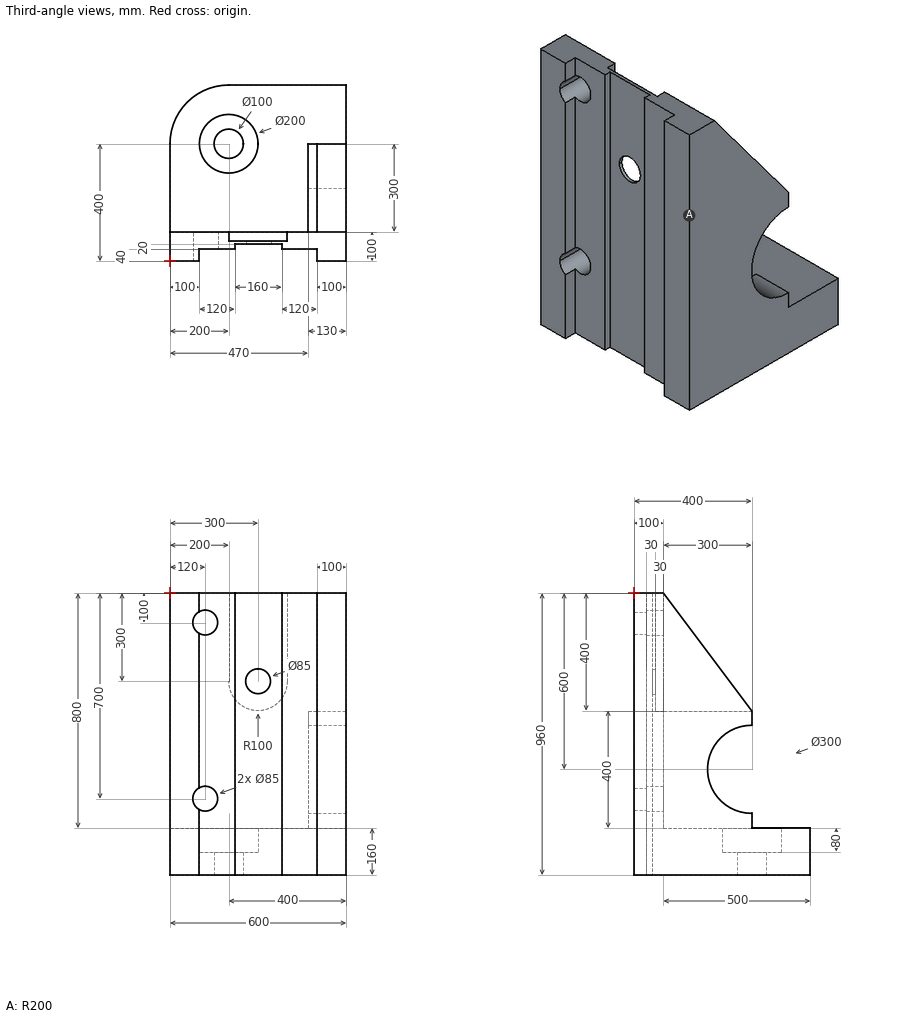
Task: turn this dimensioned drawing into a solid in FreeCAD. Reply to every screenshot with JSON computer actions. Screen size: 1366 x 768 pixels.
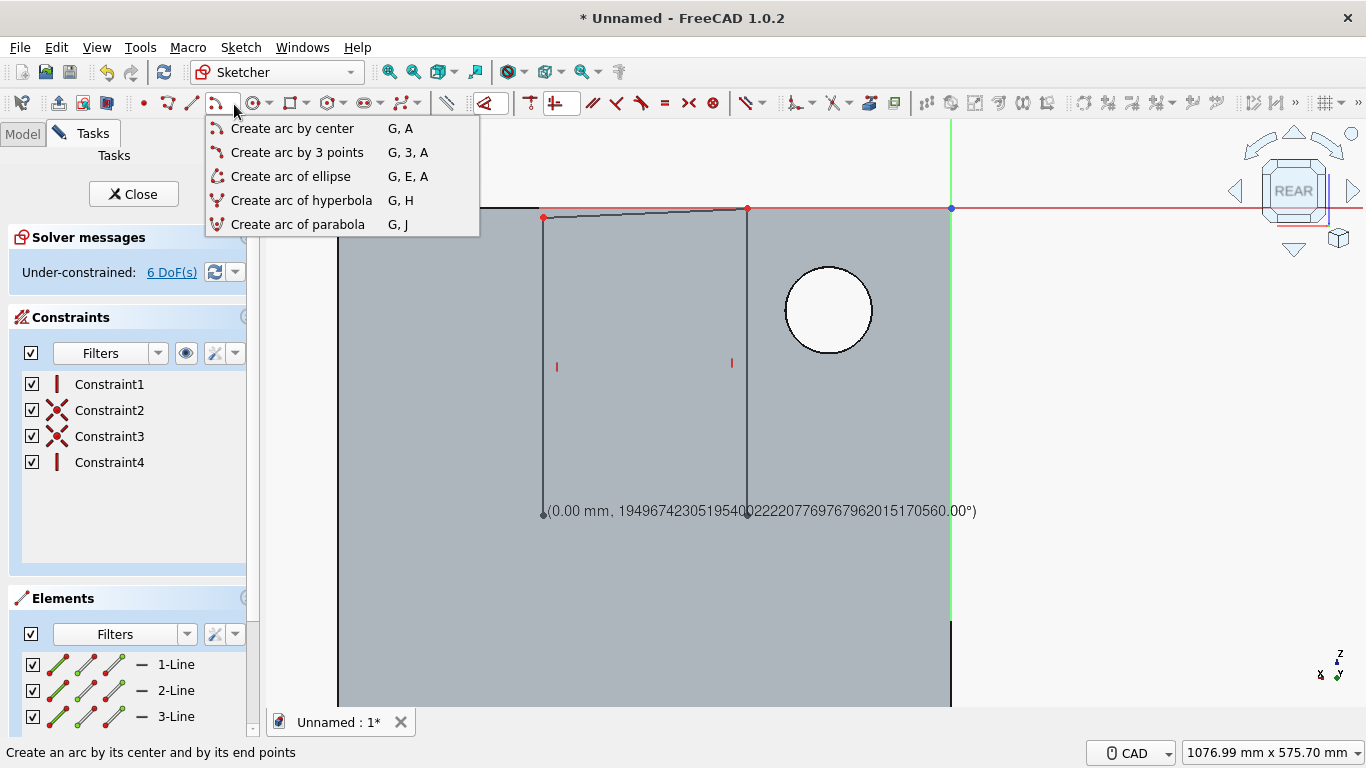
{"action": "left_click", "coordinate": [342, 152]}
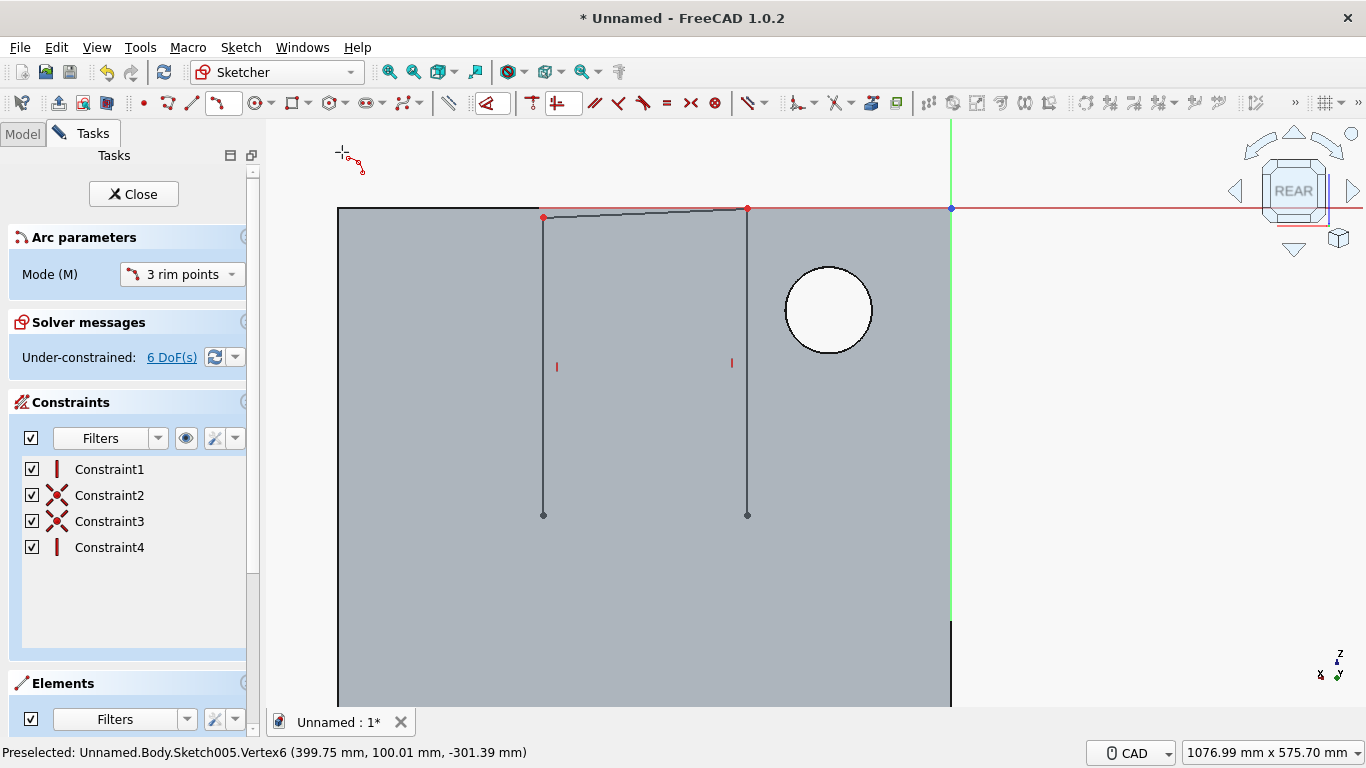
{"action": "left_click", "coordinate": [543, 516]}
{"action": "left_click", "coordinate": [747, 516]}
{"action": "left_click", "coordinate": [645, 617]}
{"action": "key", "text": "Escape"}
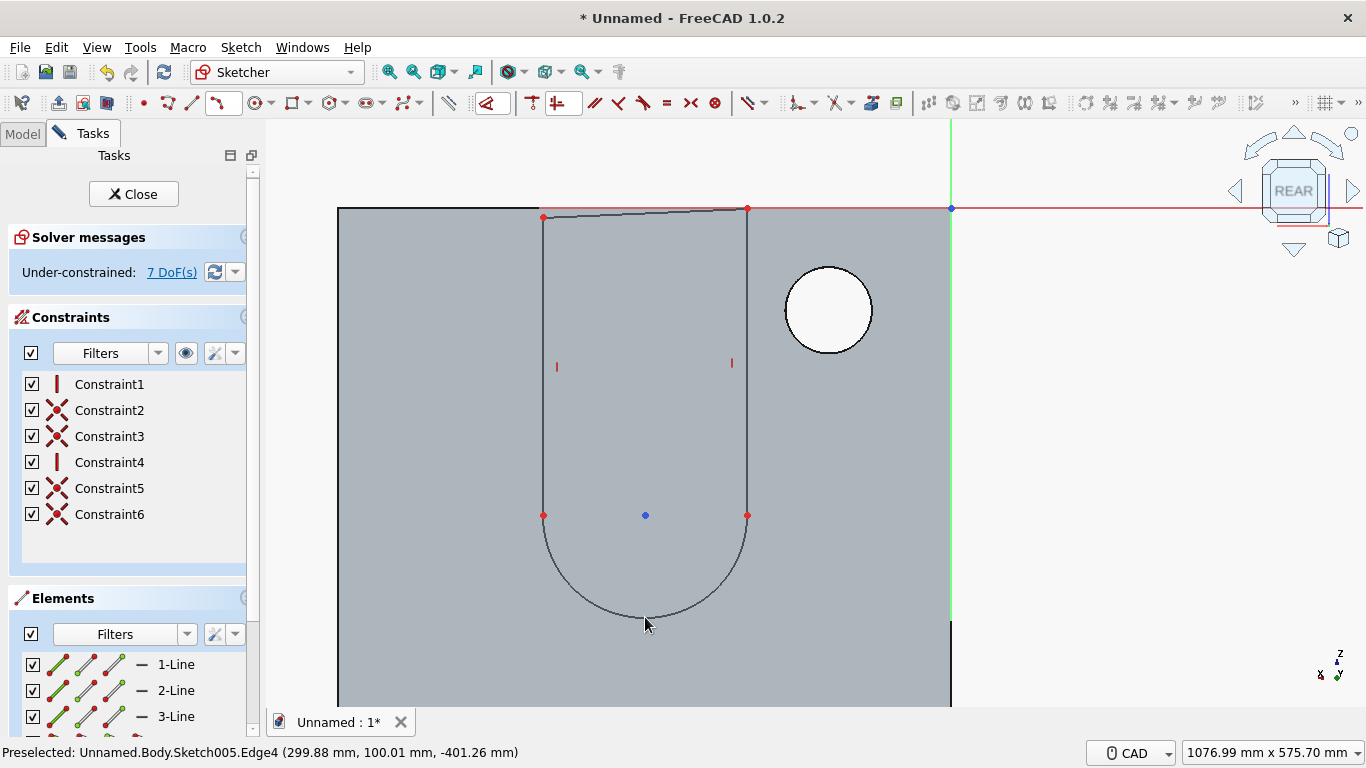
{"action": "left_click", "coordinate": [686, 212]}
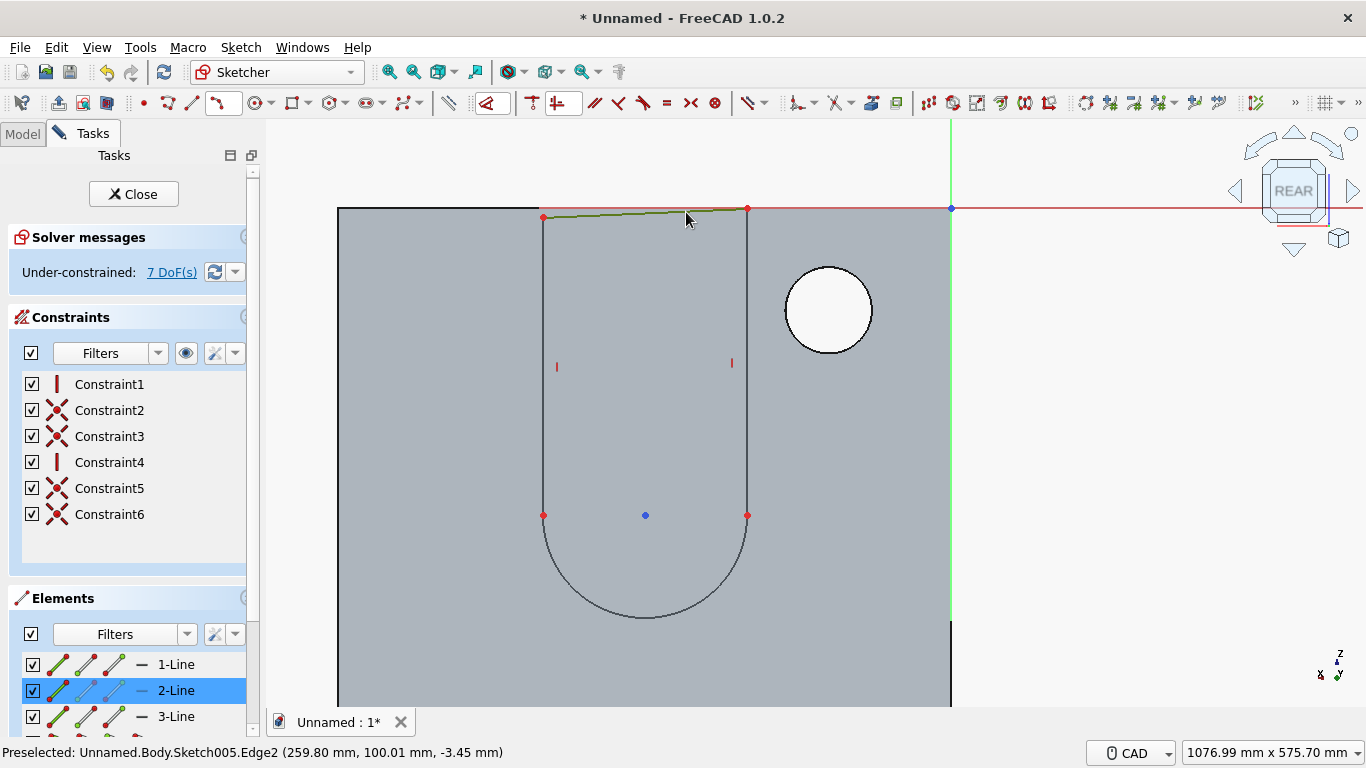
{"action": "key", "text": "h"}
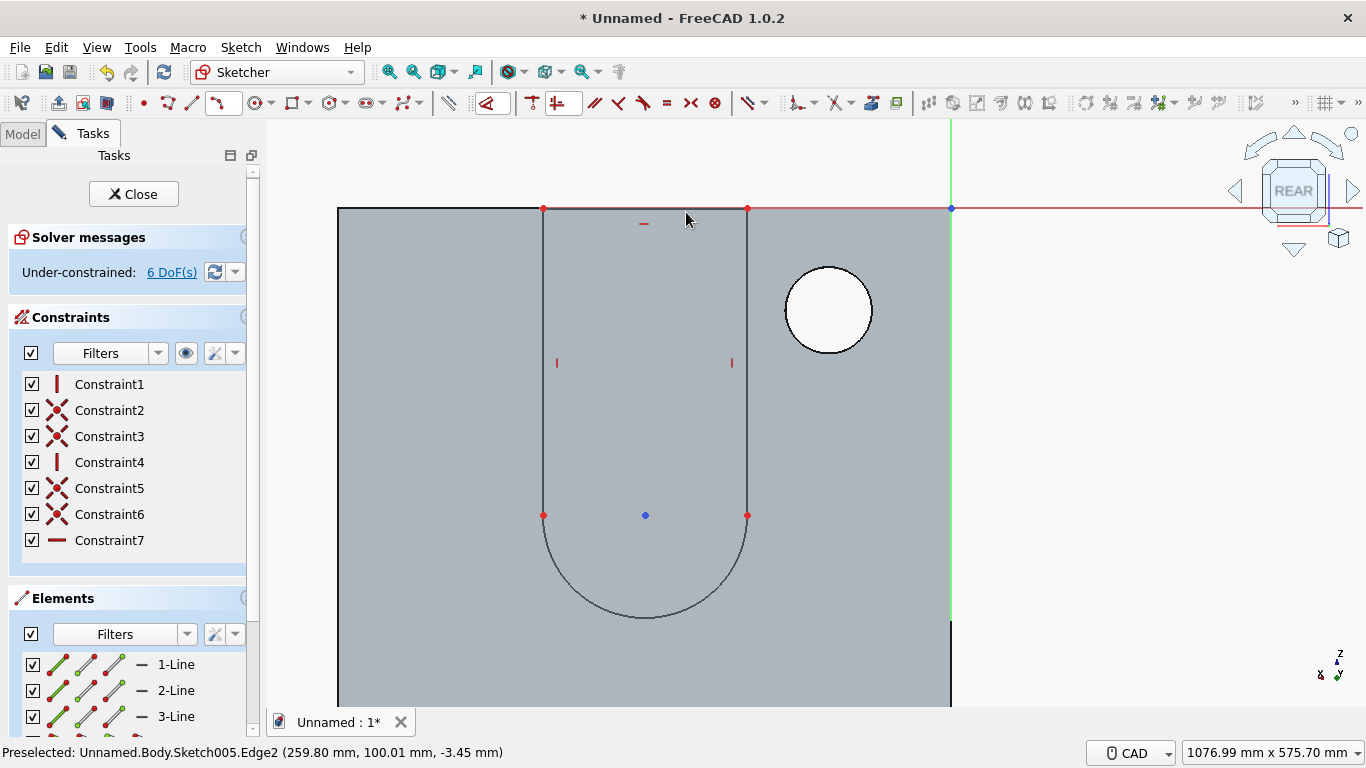
{"action": "left_click", "coordinate": [585, 599]}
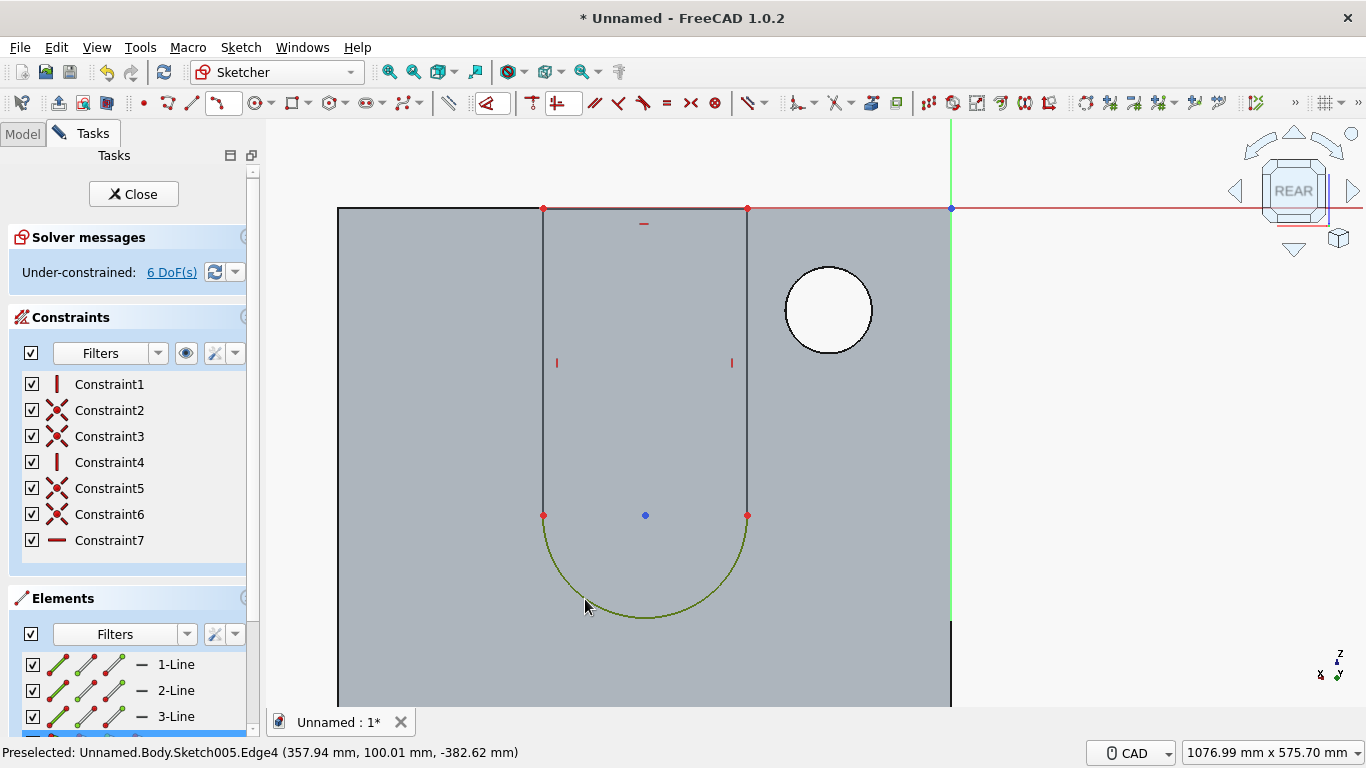
{"action": "left_click", "coordinate": [504, 104]}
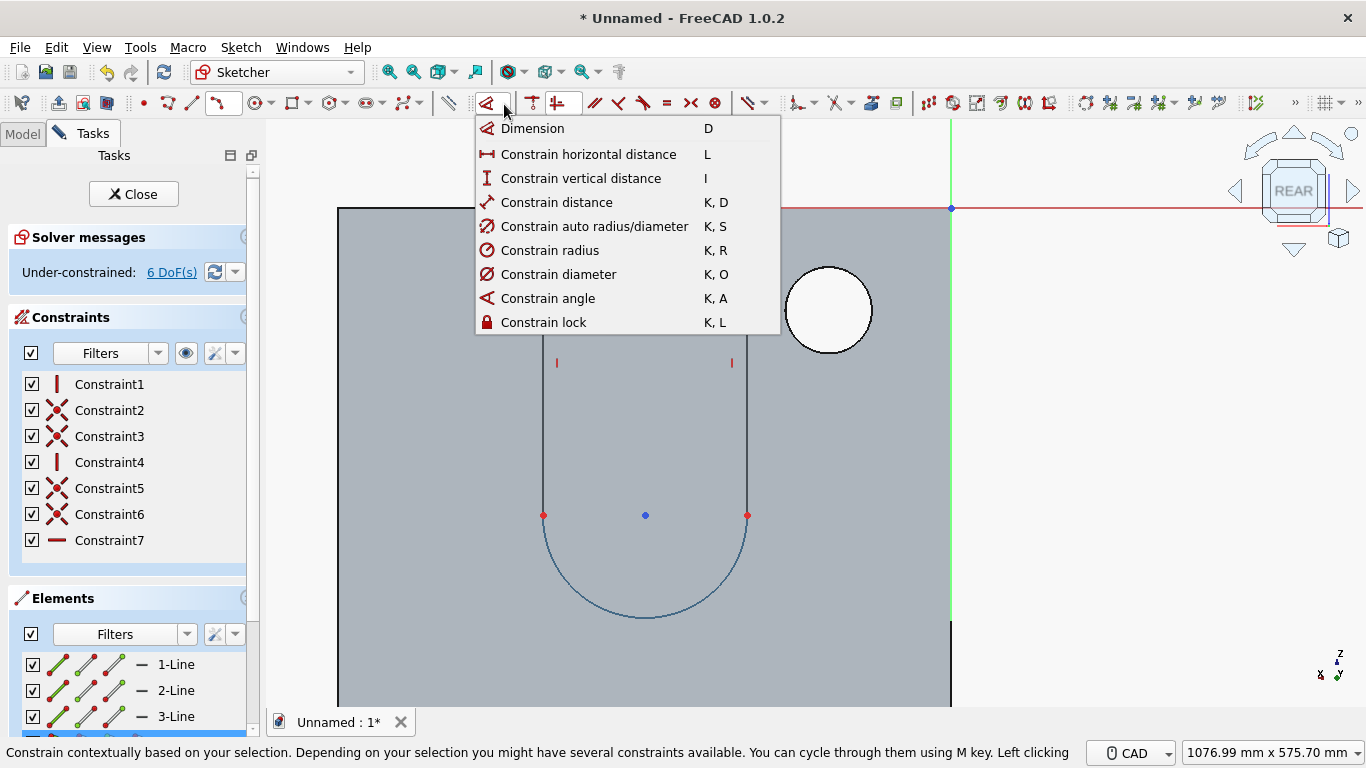
{"action": "left_click", "coordinate": [628, 250]}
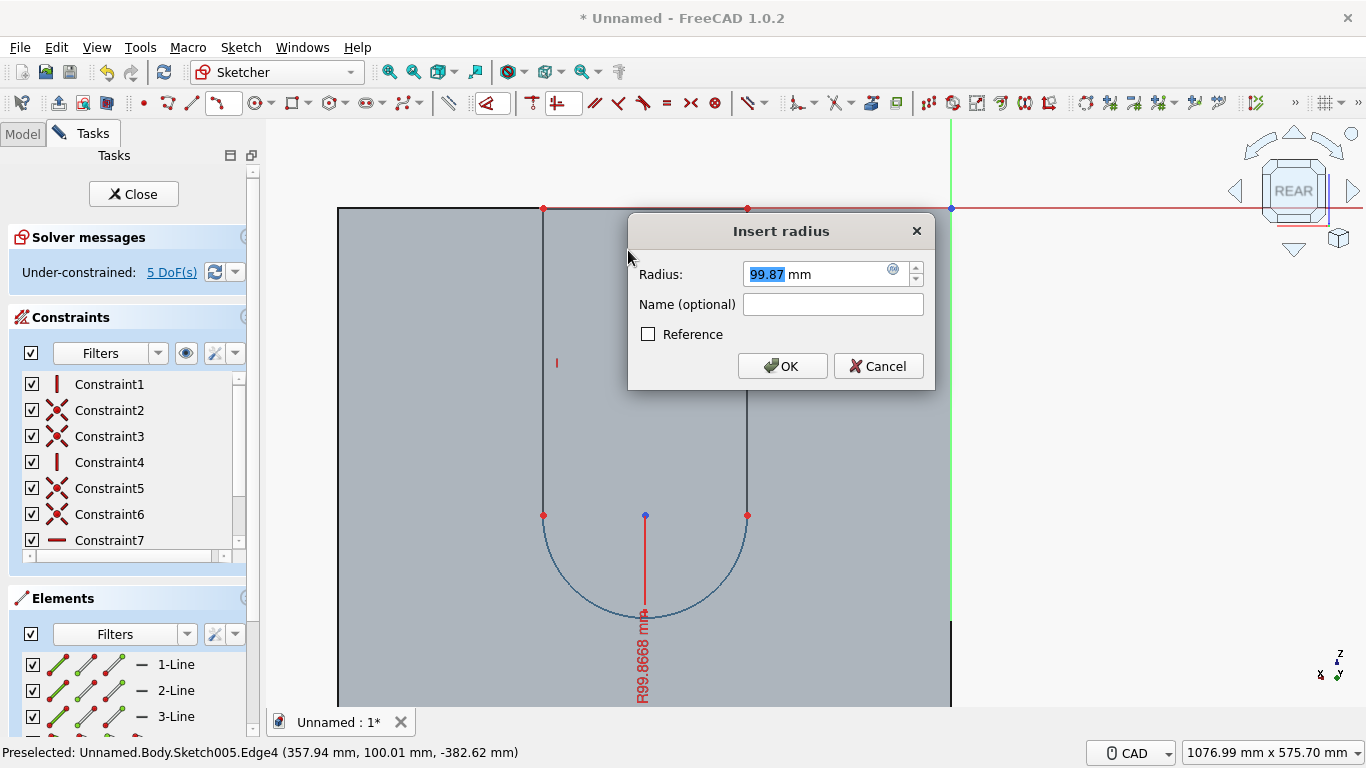
{"action": "type", "text": "100"}
{"action": "key", "text": "Return"}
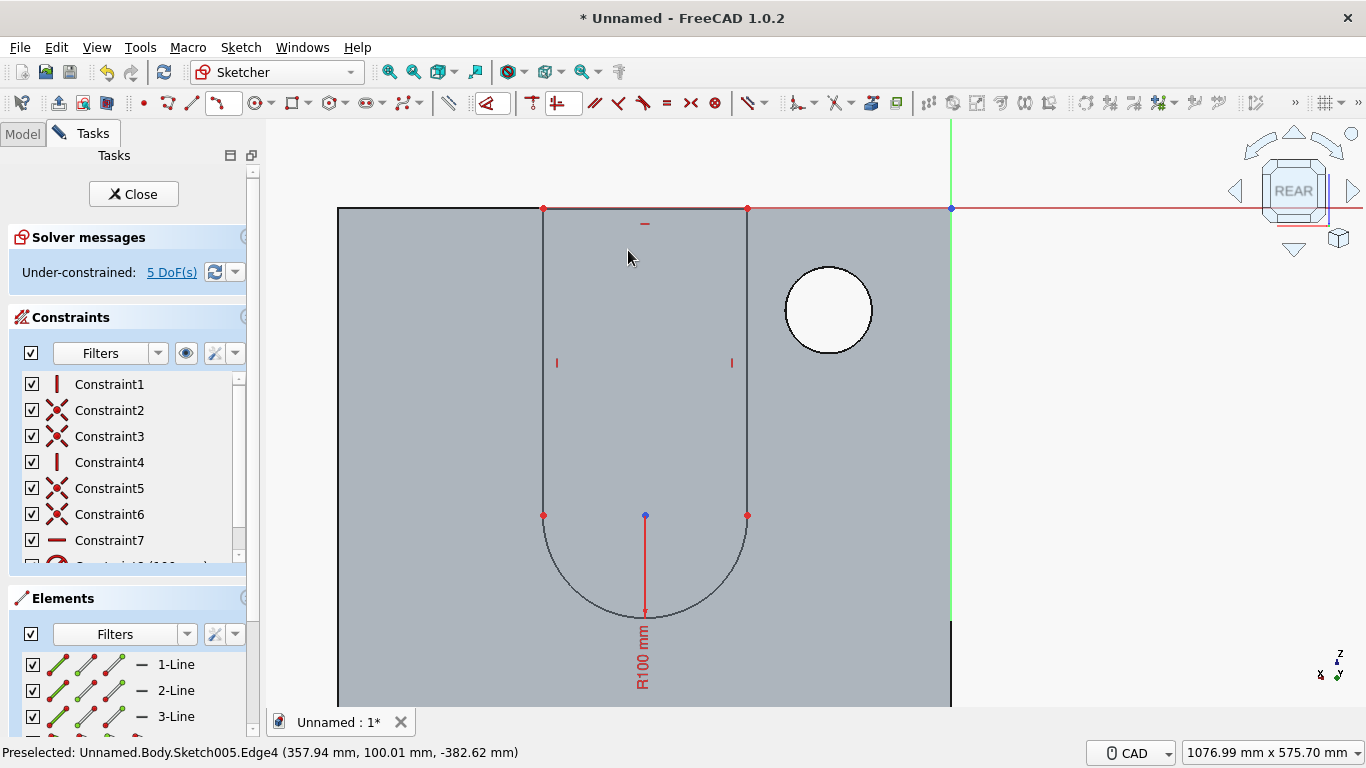
{"action": "left_click", "coordinate": [747, 209]}